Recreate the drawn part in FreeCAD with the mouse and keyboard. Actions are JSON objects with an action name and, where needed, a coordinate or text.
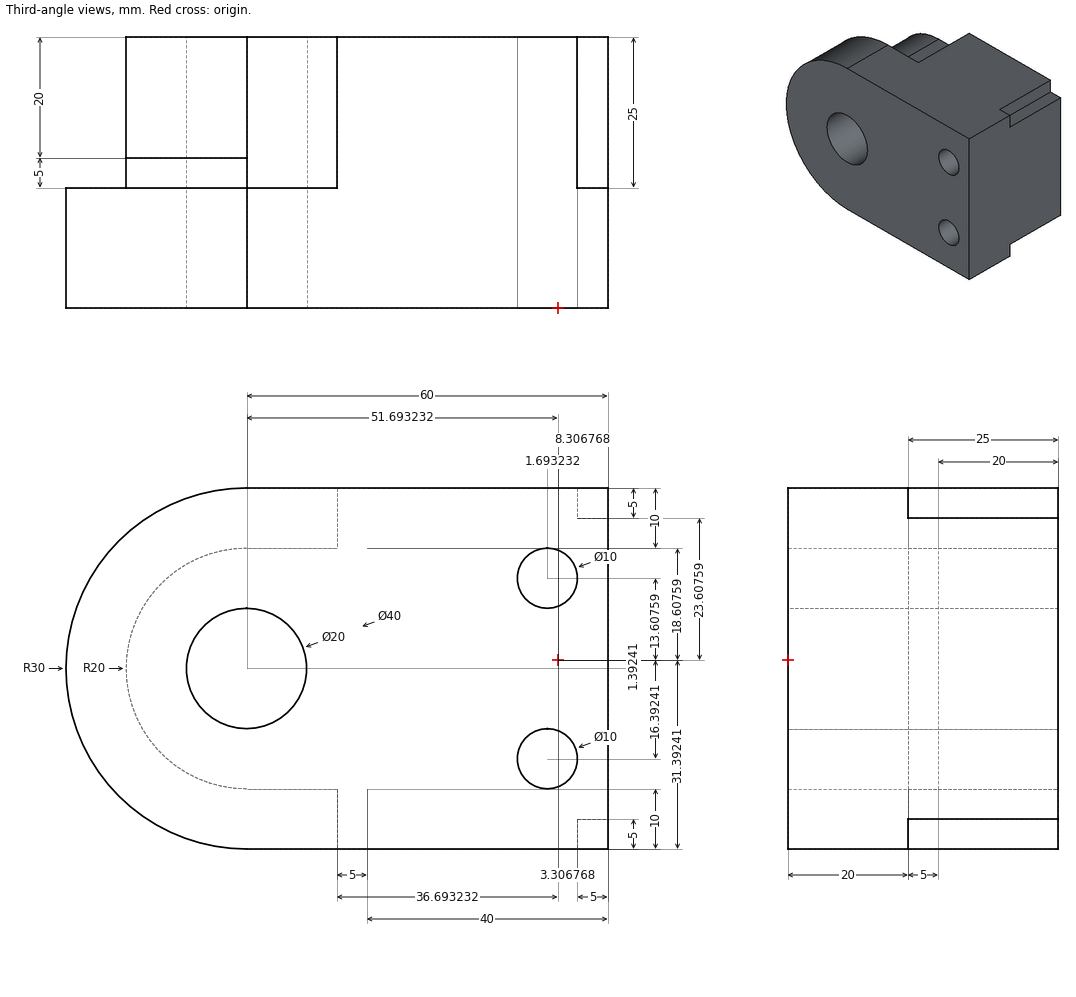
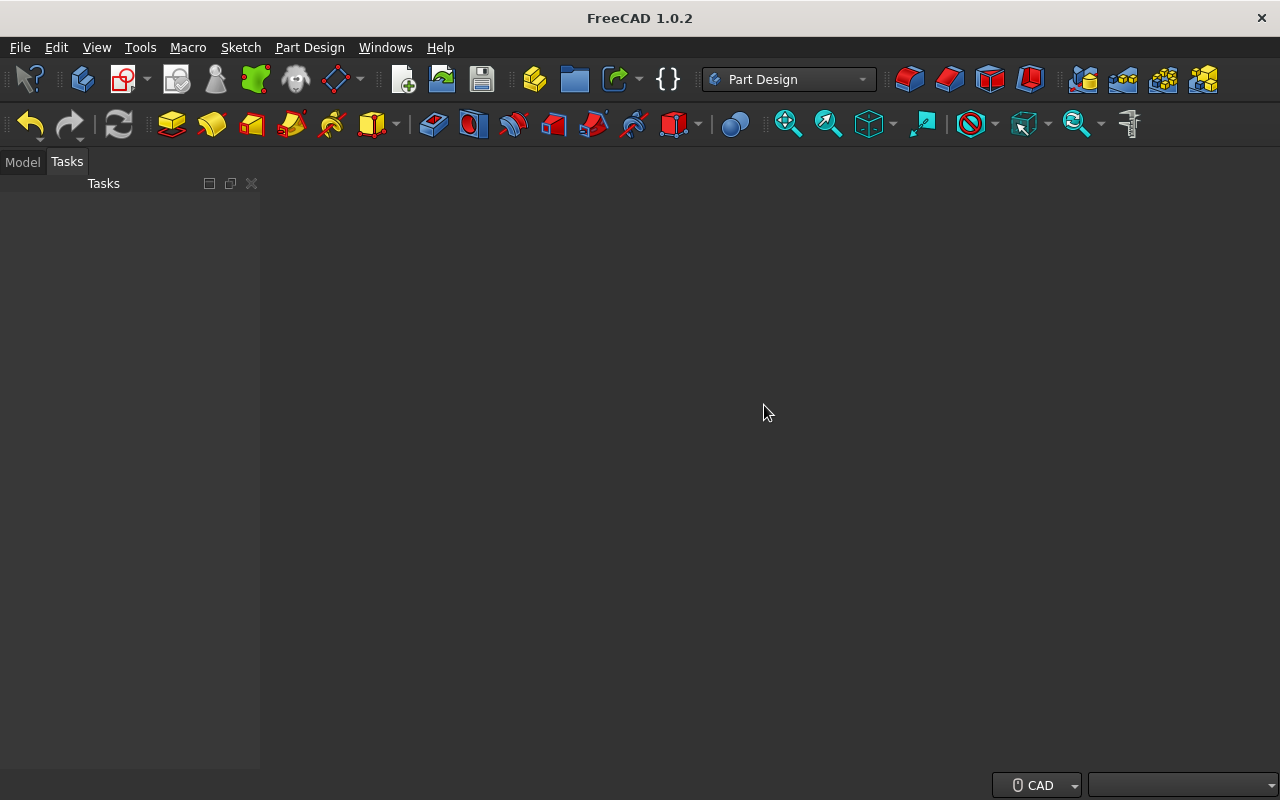
{"action": "left_click", "coordinate": [402, 80]}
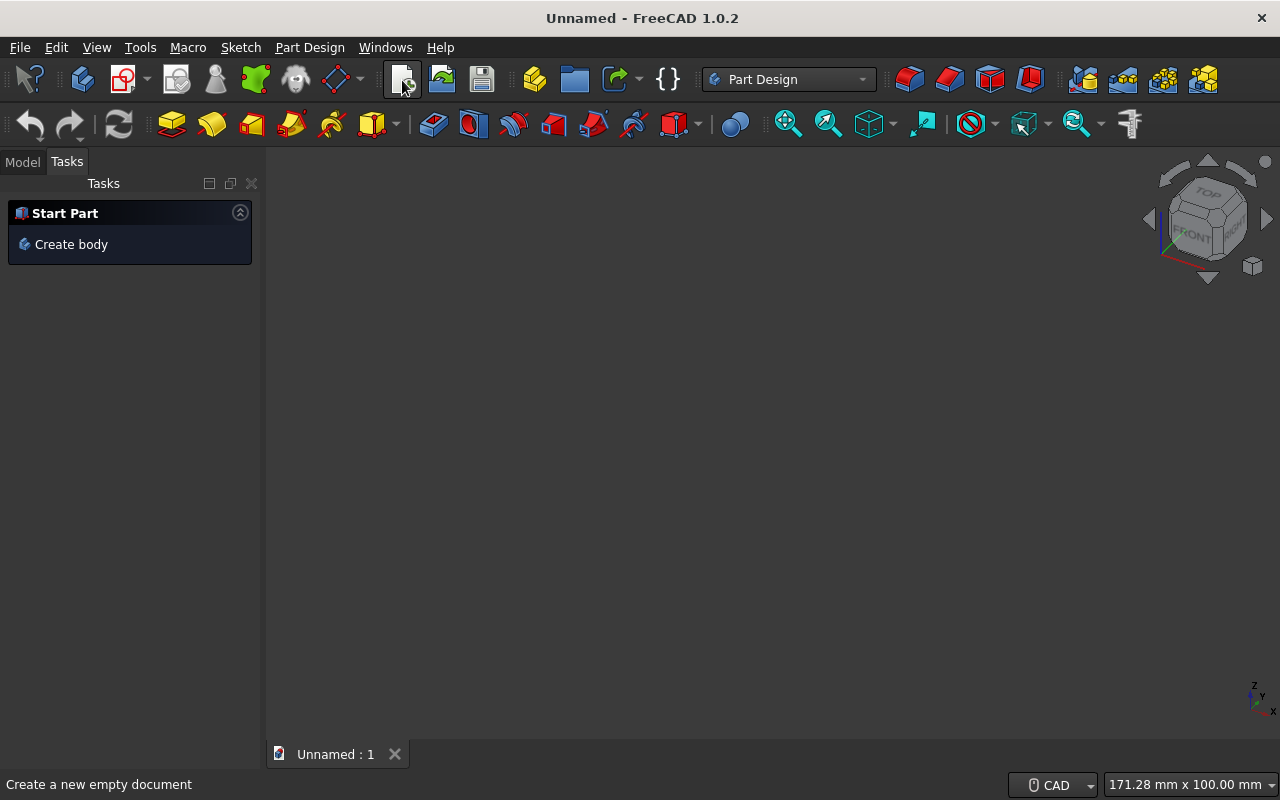
{"action": "left_click", "coordinate": [124, 80]}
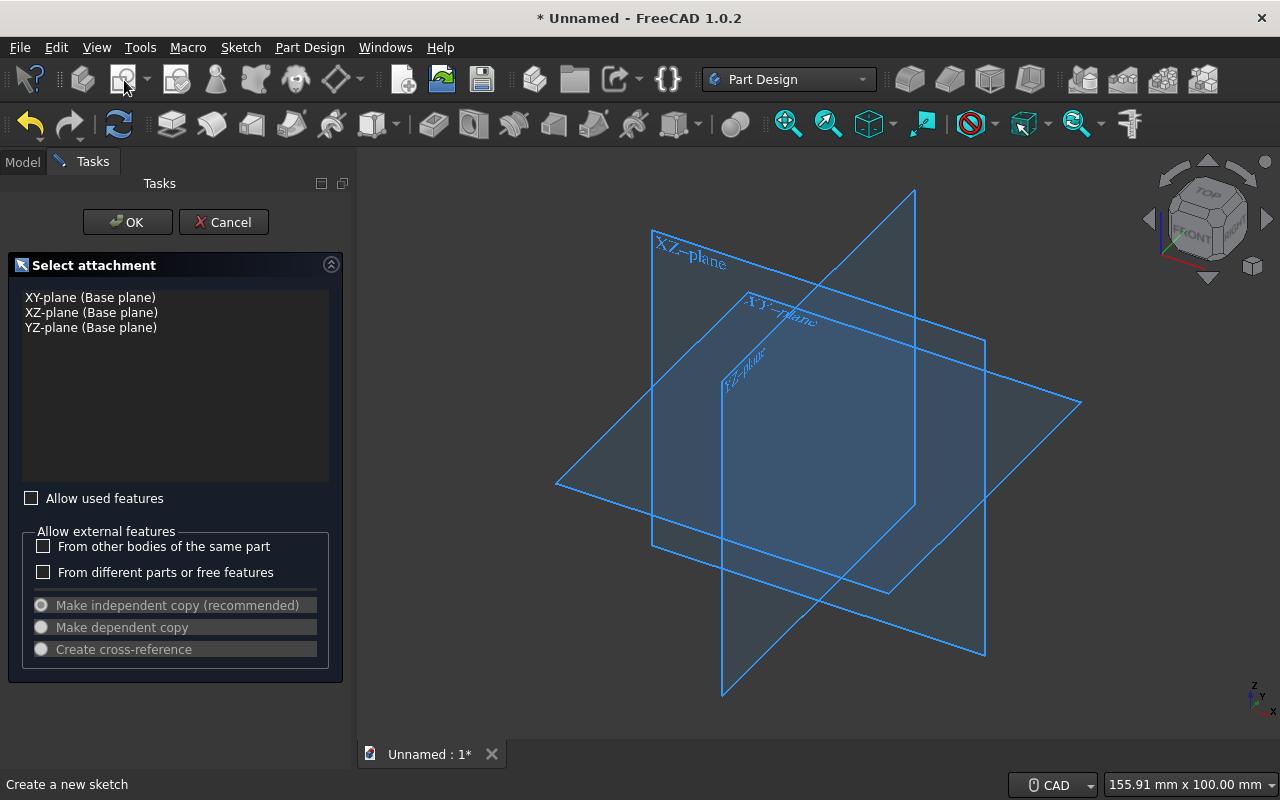
{"action": "left_click", "coordinate": [82, 312]}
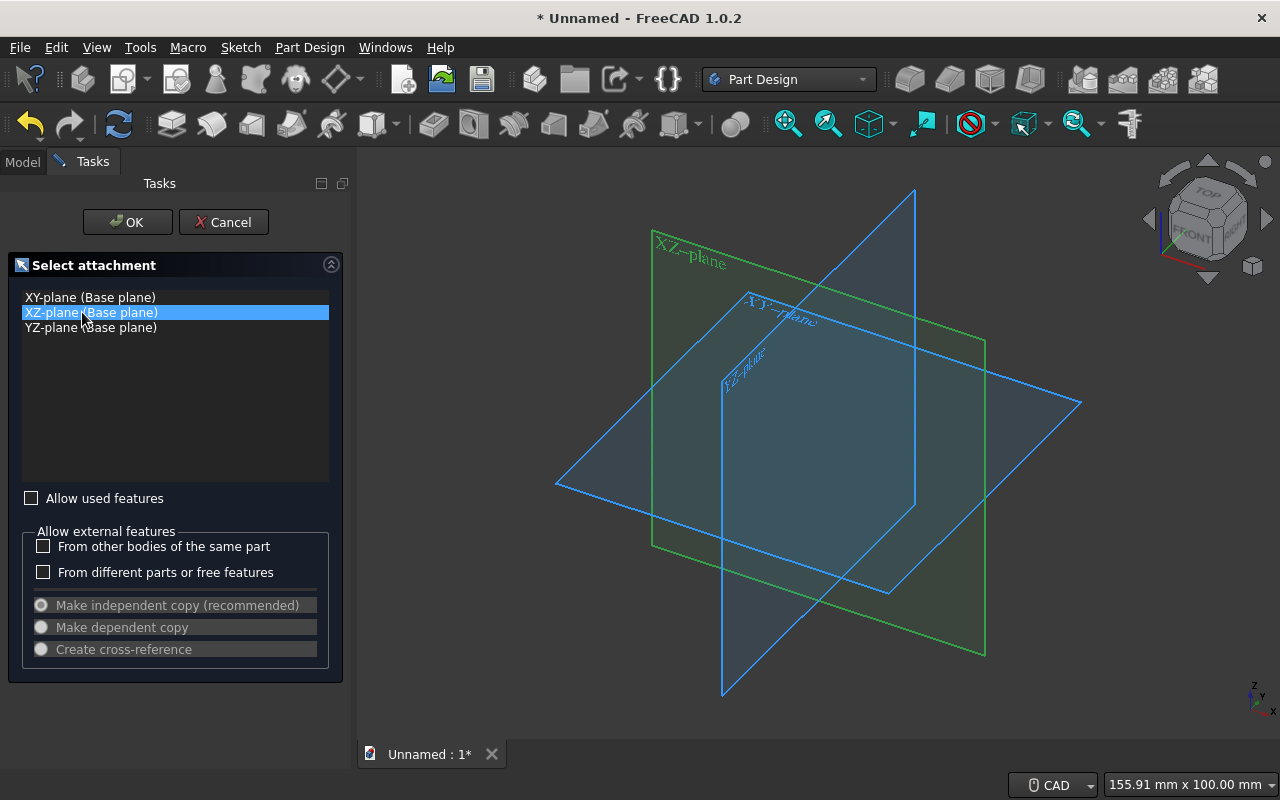
{"action": "left_click", "coordinate": [128, 222]}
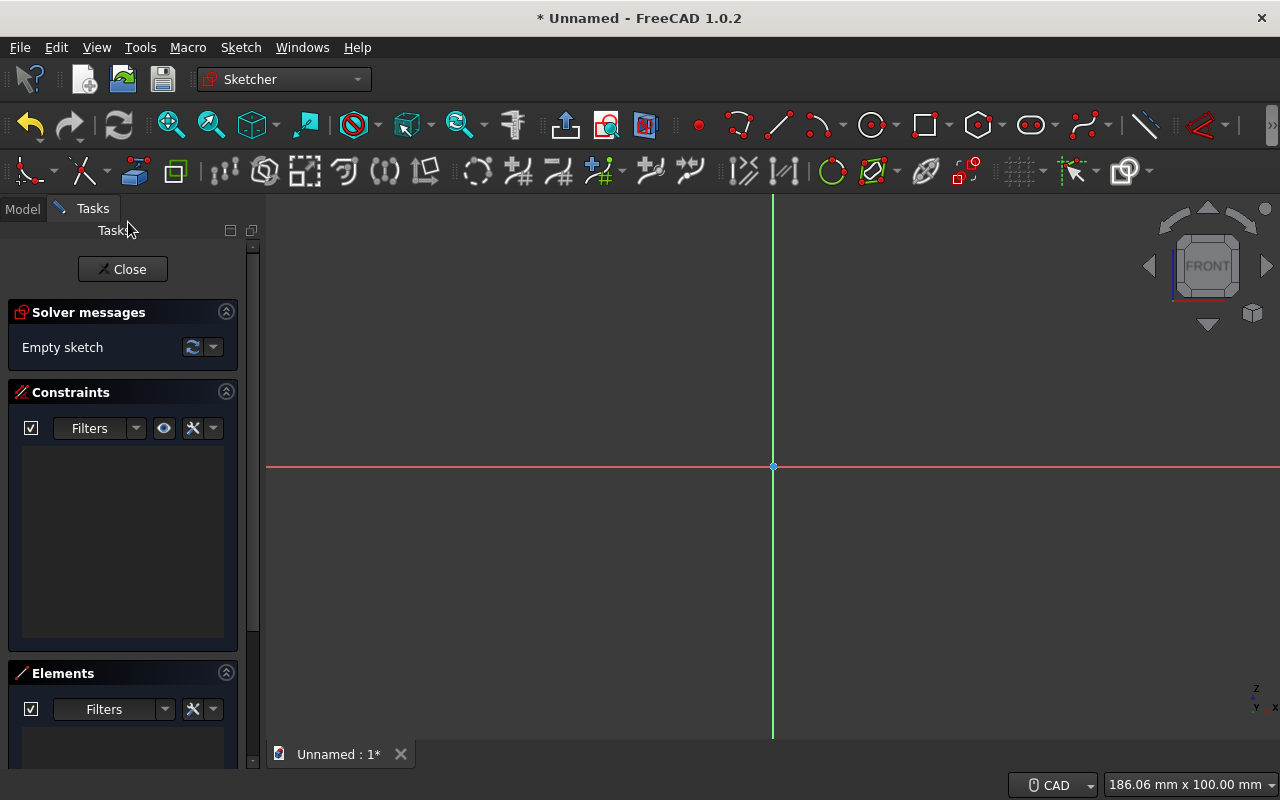
{"action": "key", "text": "g m"}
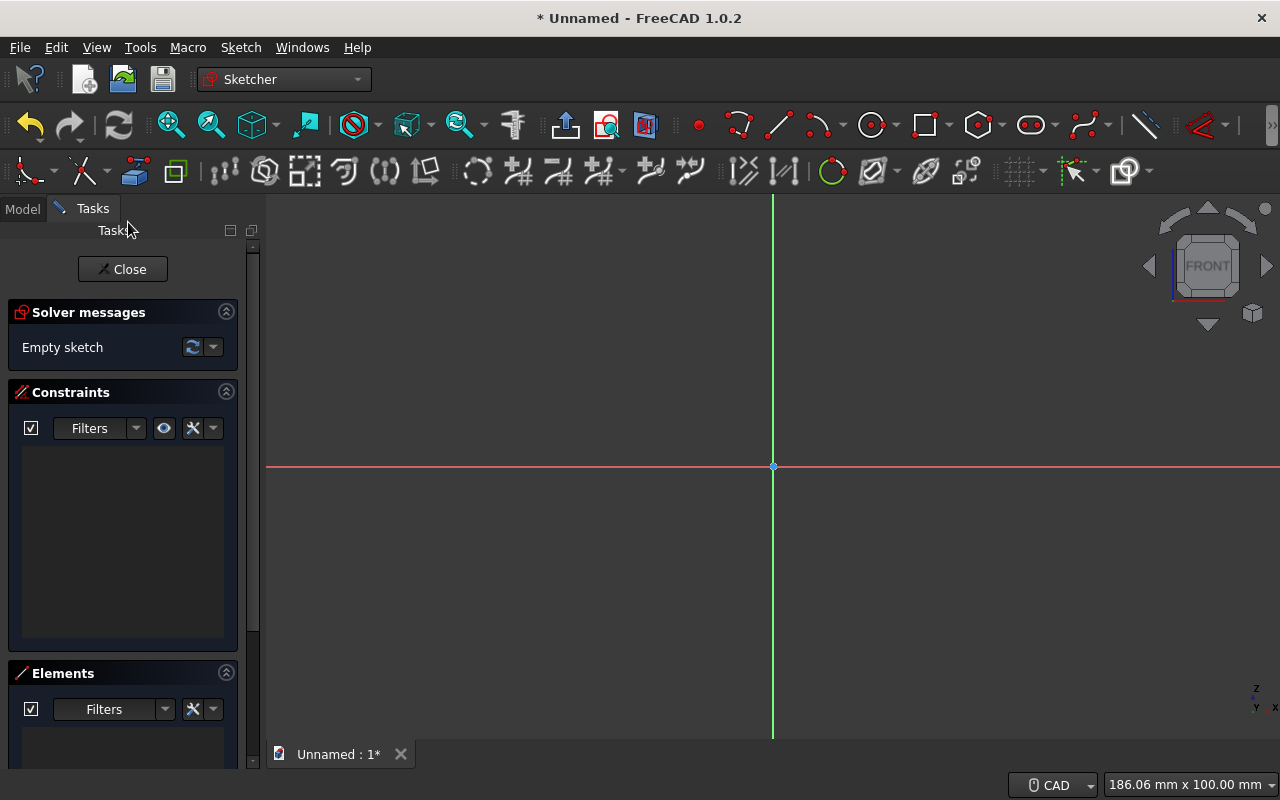
{"action": "left_click", "coordinate": [491, 311]}
{"action": "left_click", "coordinate": [818, 311]}
{"action": "left_click", "coordinate": [818, 638]}
{"action": "left_click", "coordinate": [491, 638]}
{"action": "right_click", "coordinate": [491, 638]}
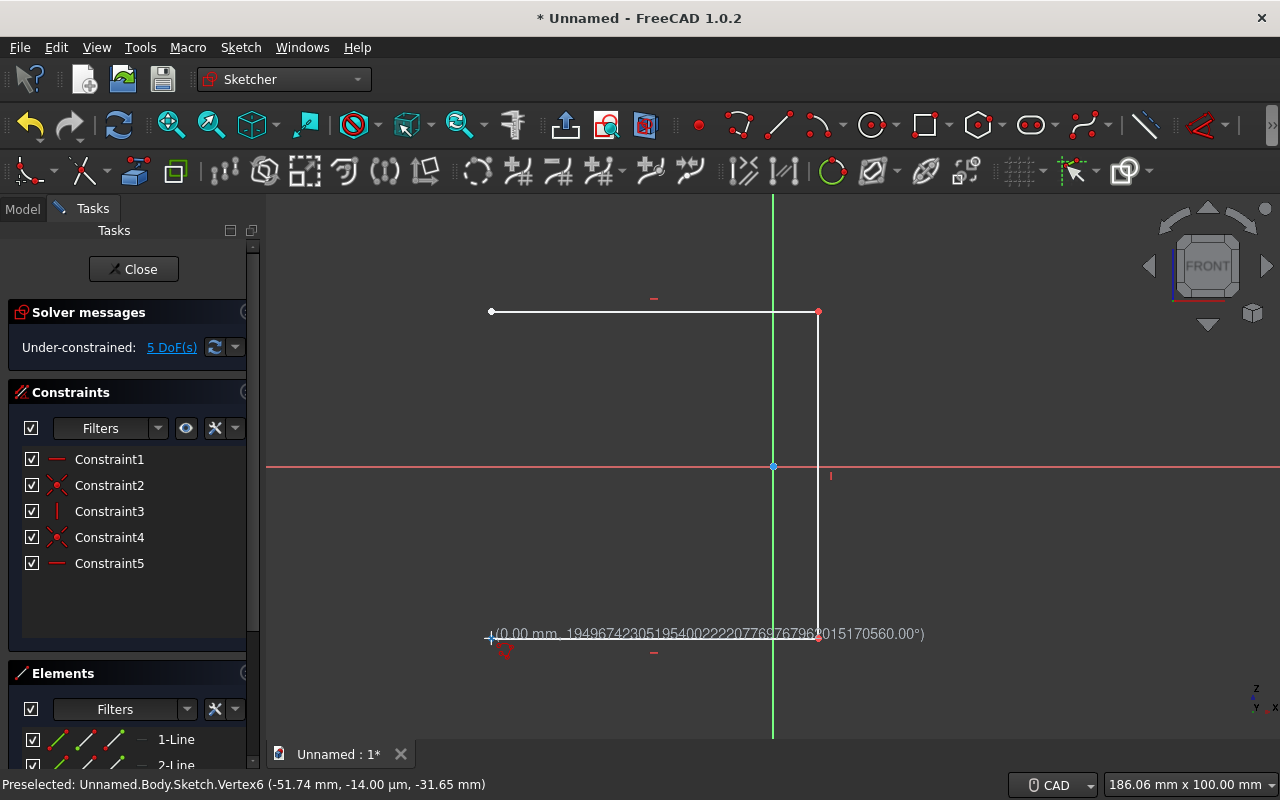
{"action": "key", "text": "g 3 a"}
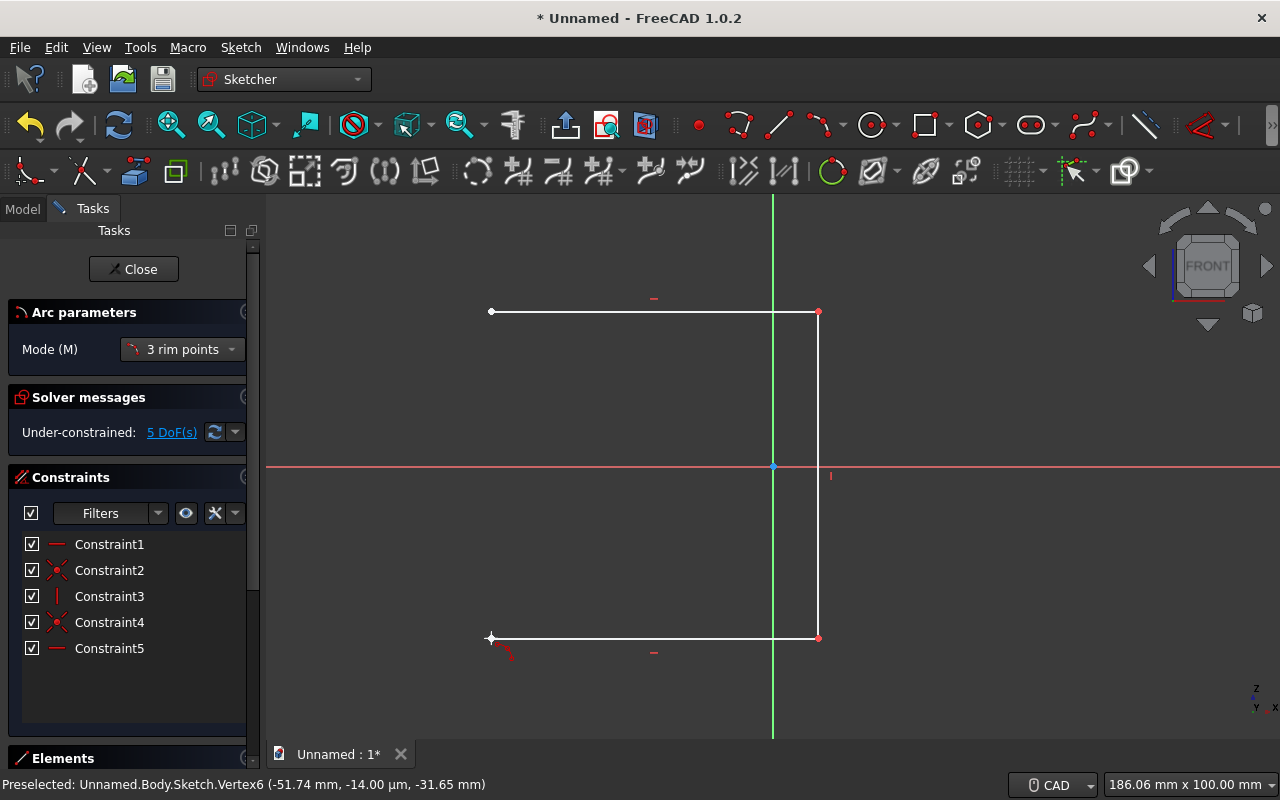
{"action": "left_click", "coordinate": [491, 639]}
{"action": "left_click", "coordinate": [491, 312]}
{"action": "left_click", "coordinate": [336, 424]}
{"action": "key", "text": "Escape"}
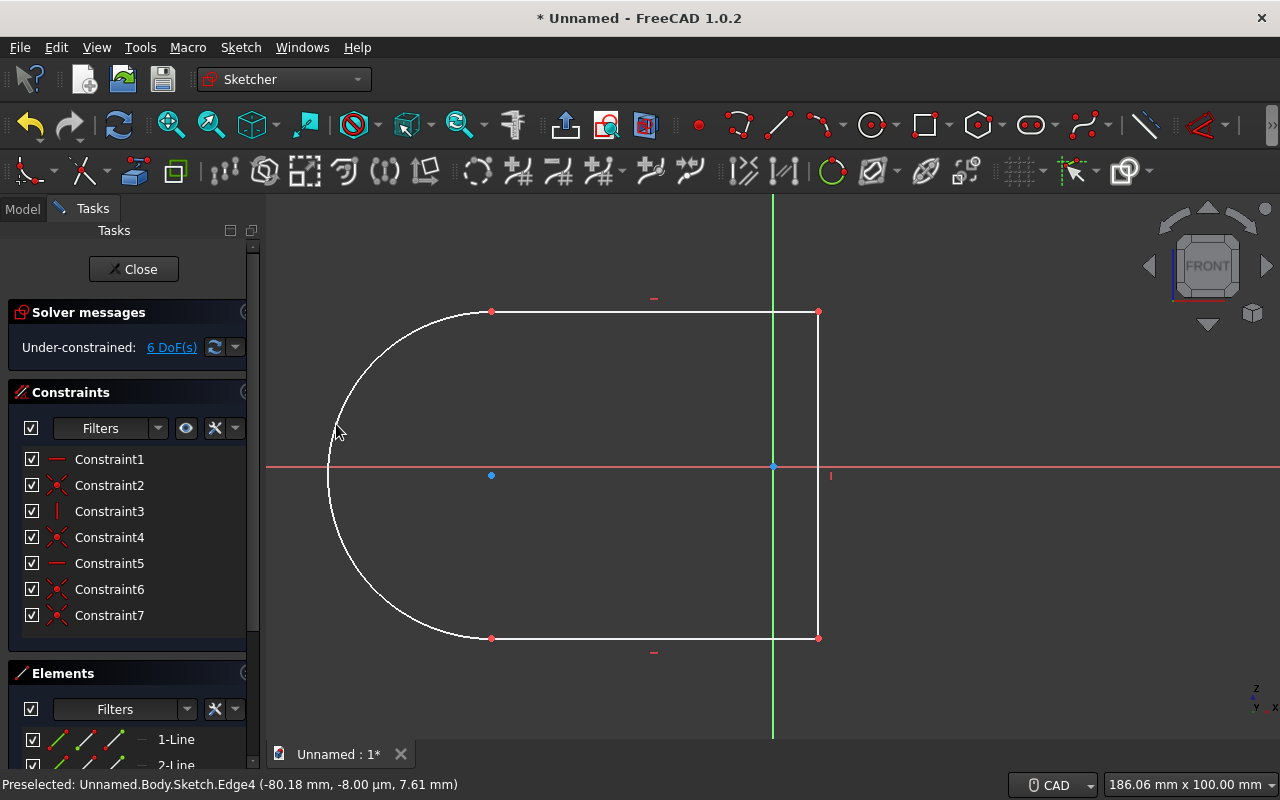
{"action": "left_click", "coordinate": [589, 312]}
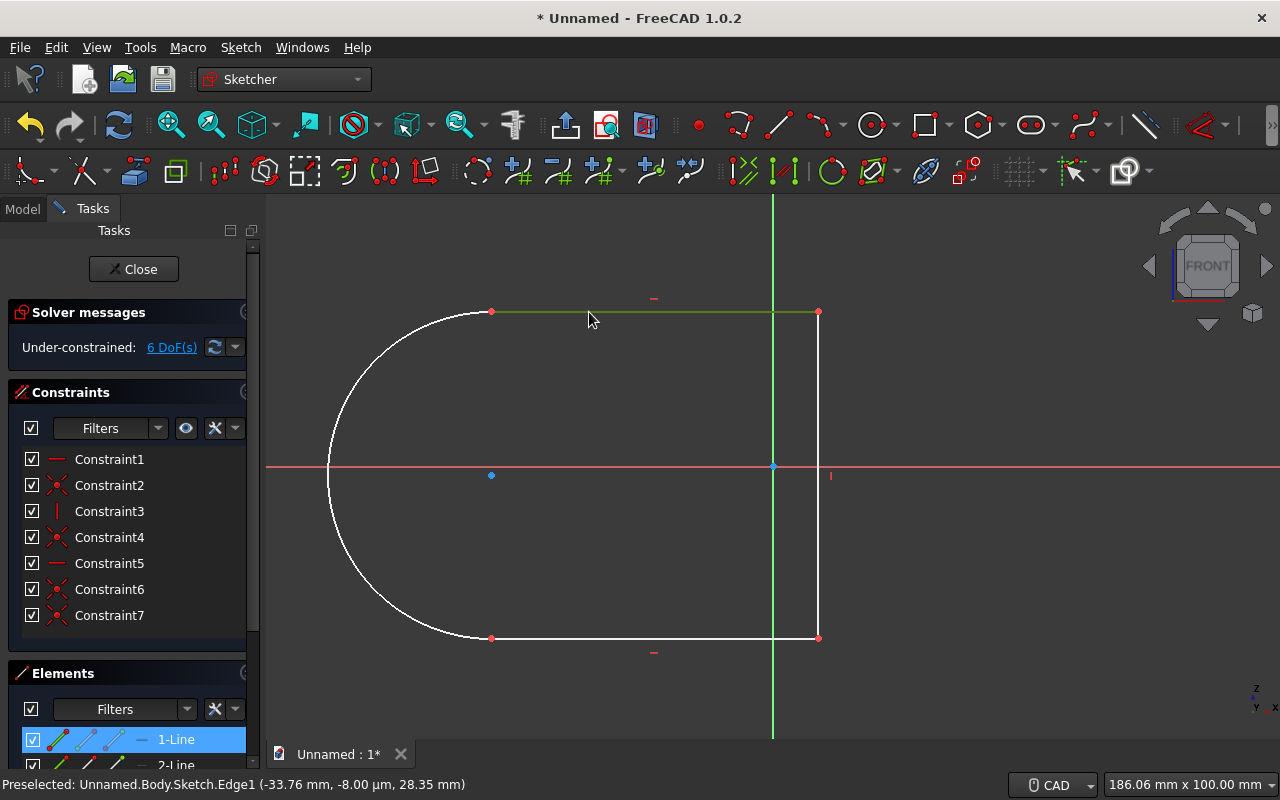
{"action": "left_click", "coordinate": [359, 380]}